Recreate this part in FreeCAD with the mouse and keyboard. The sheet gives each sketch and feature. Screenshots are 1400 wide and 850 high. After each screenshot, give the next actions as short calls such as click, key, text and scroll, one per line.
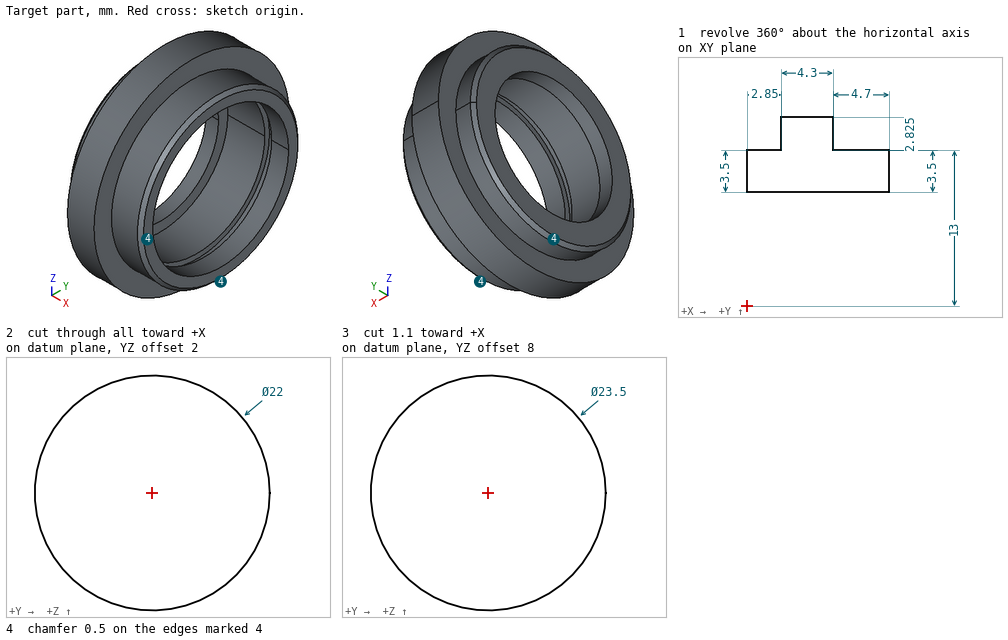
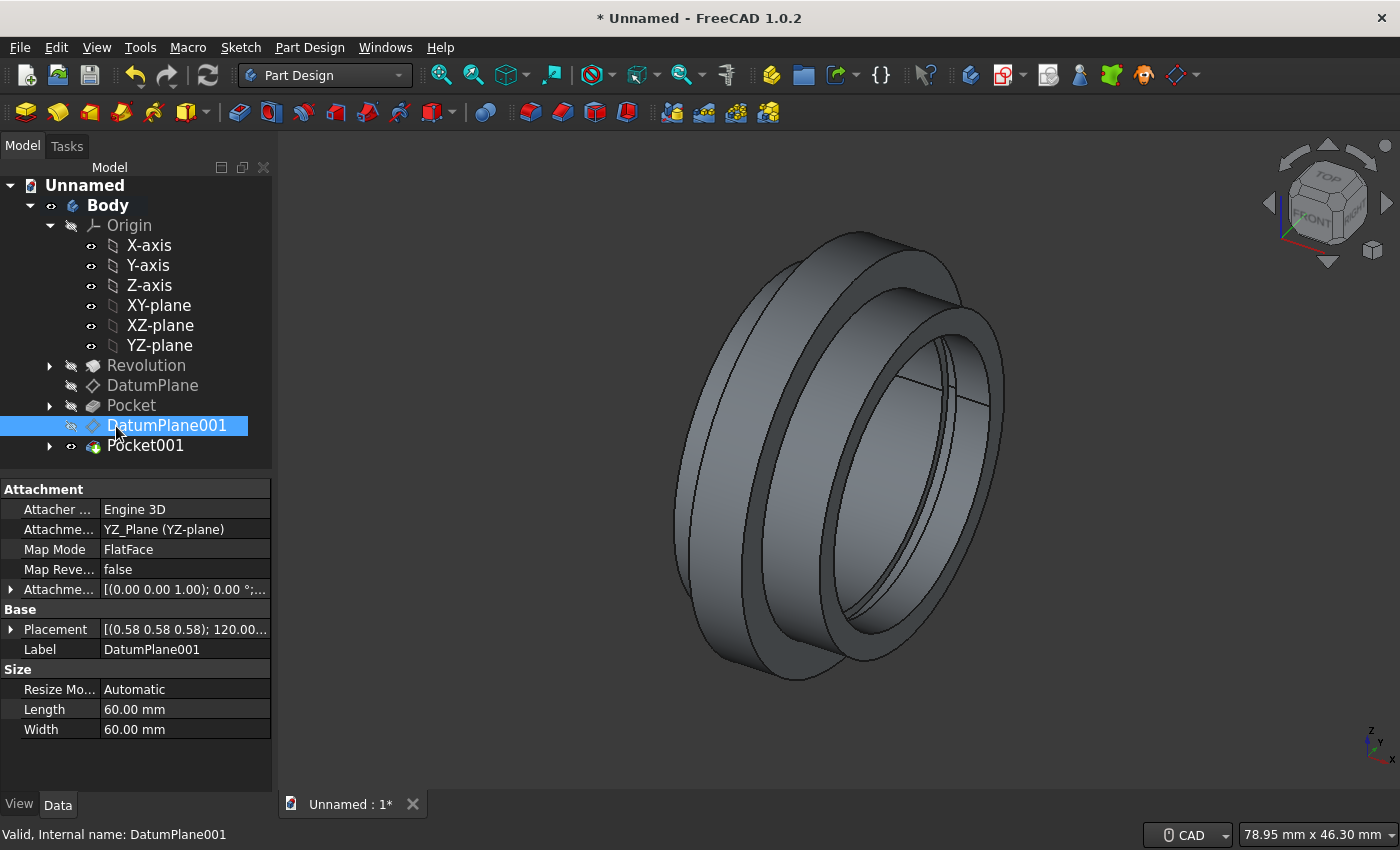
click(820, 575)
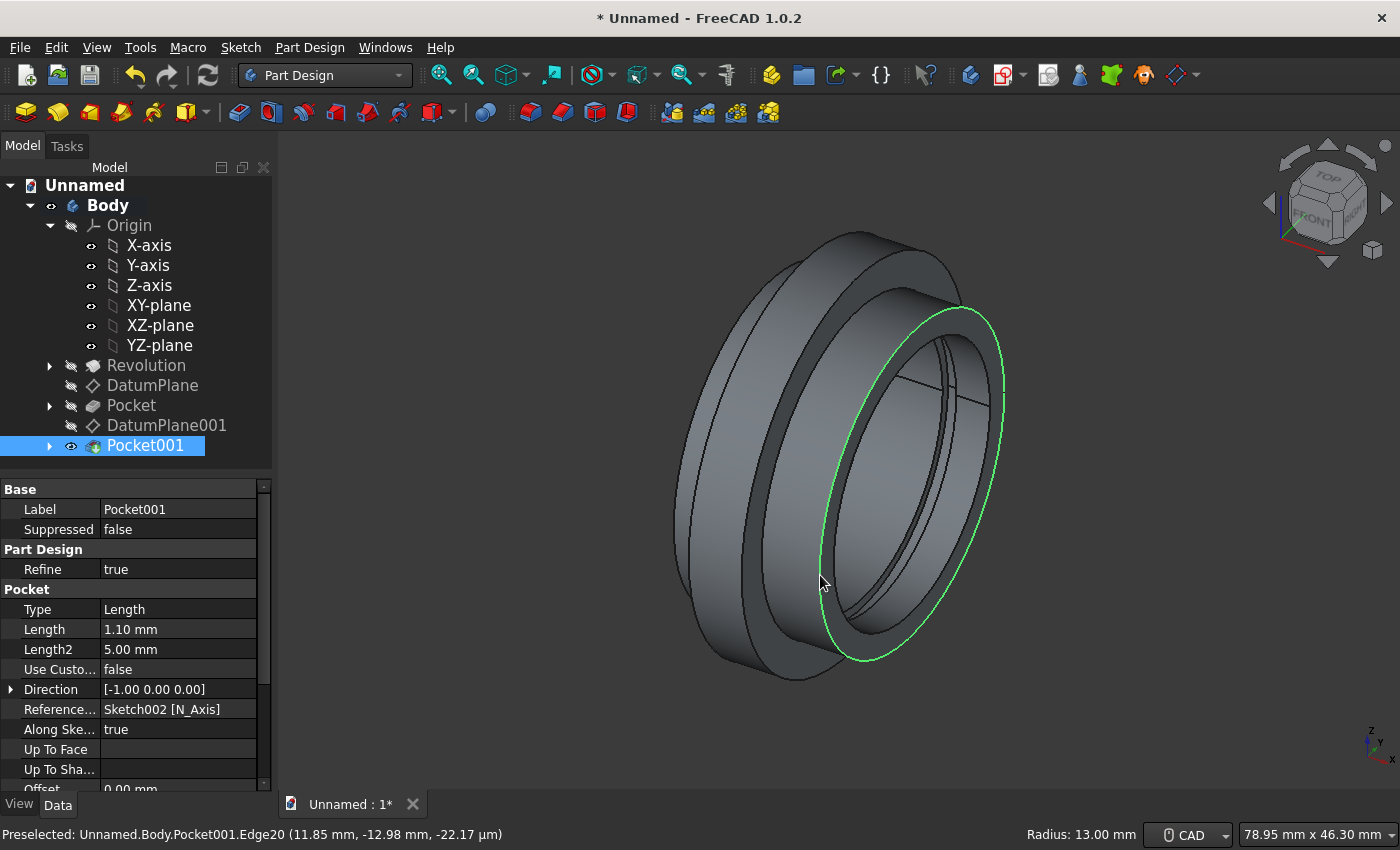
key(0)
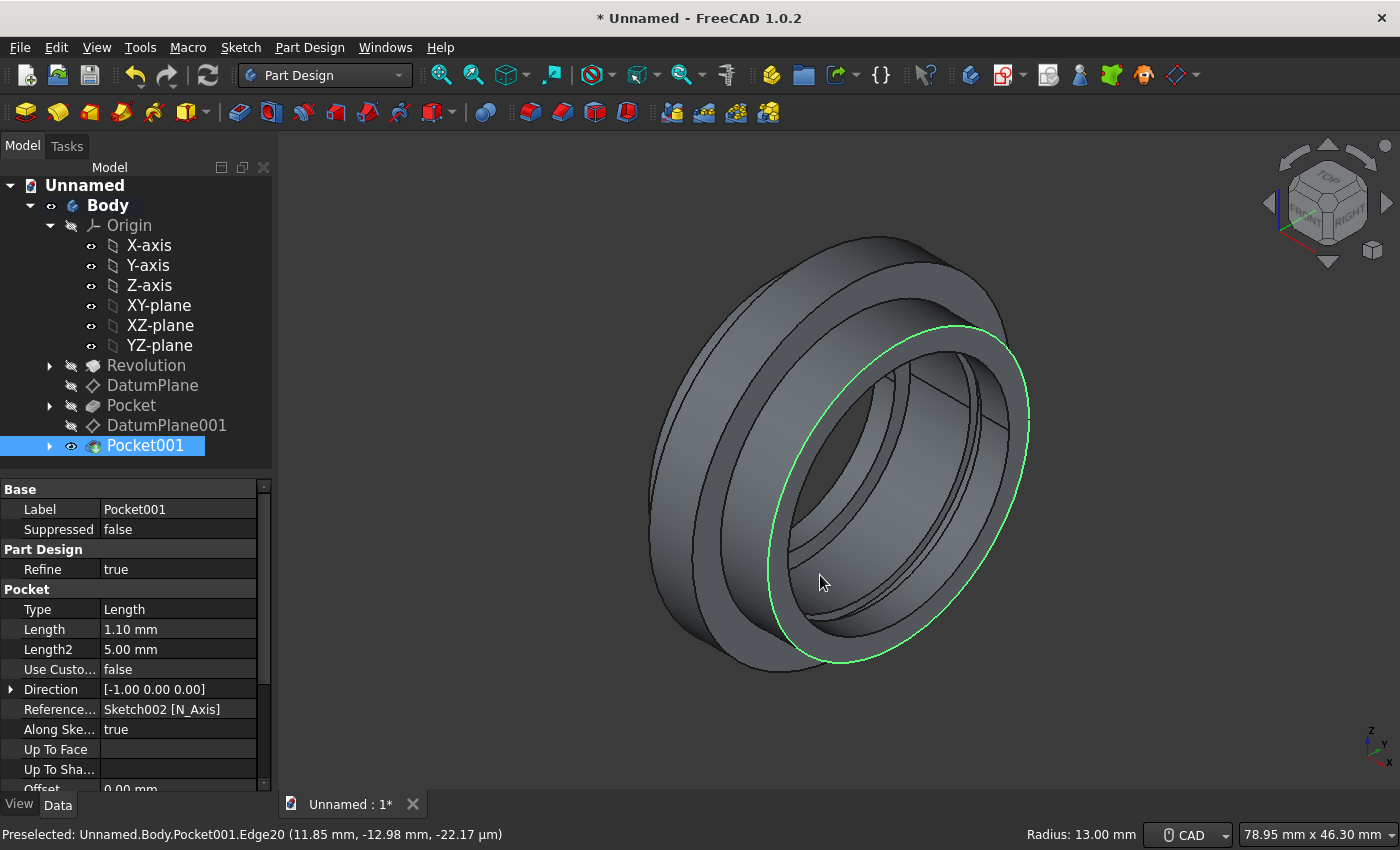
key(2)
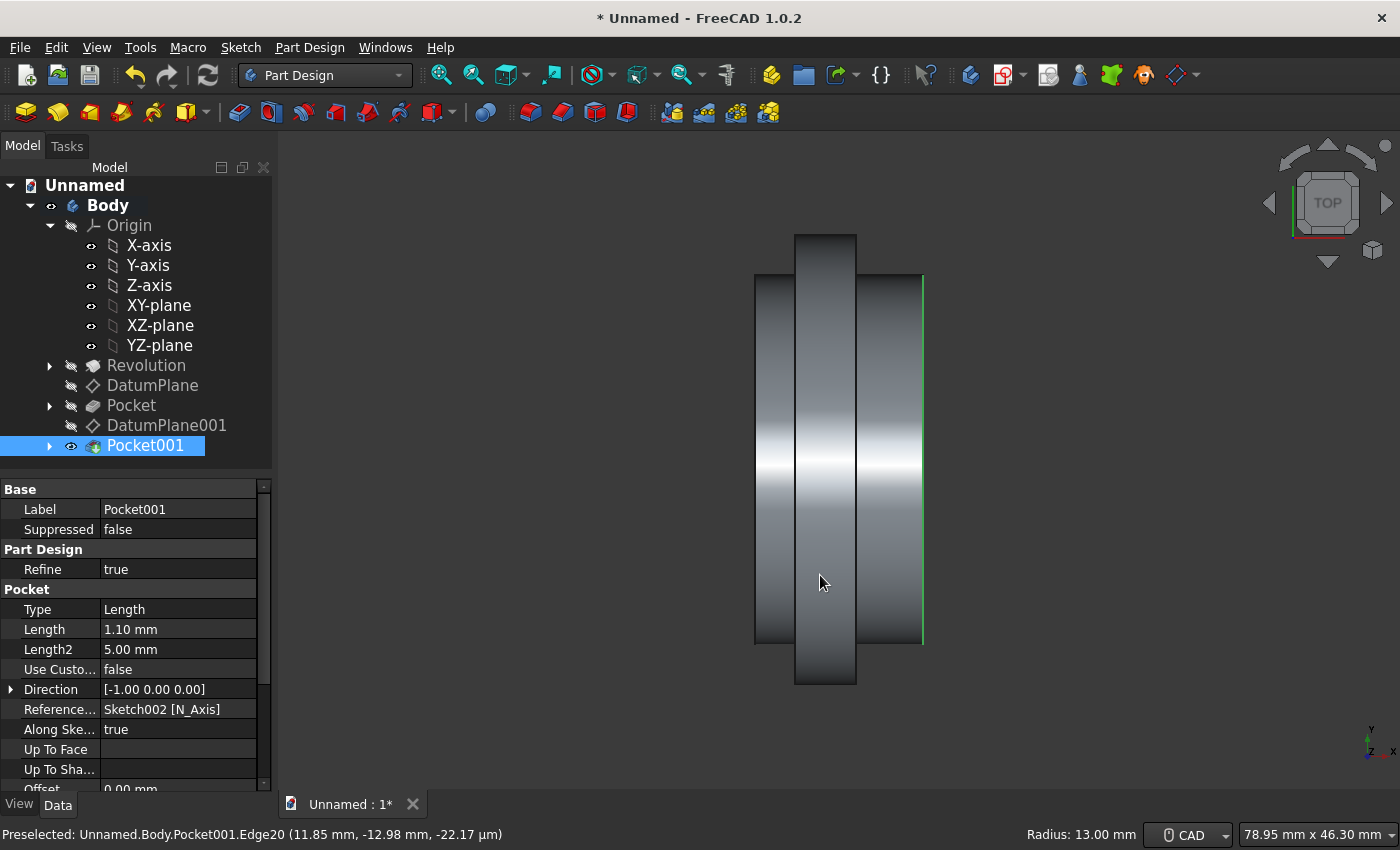
click(755, 608, ctrl)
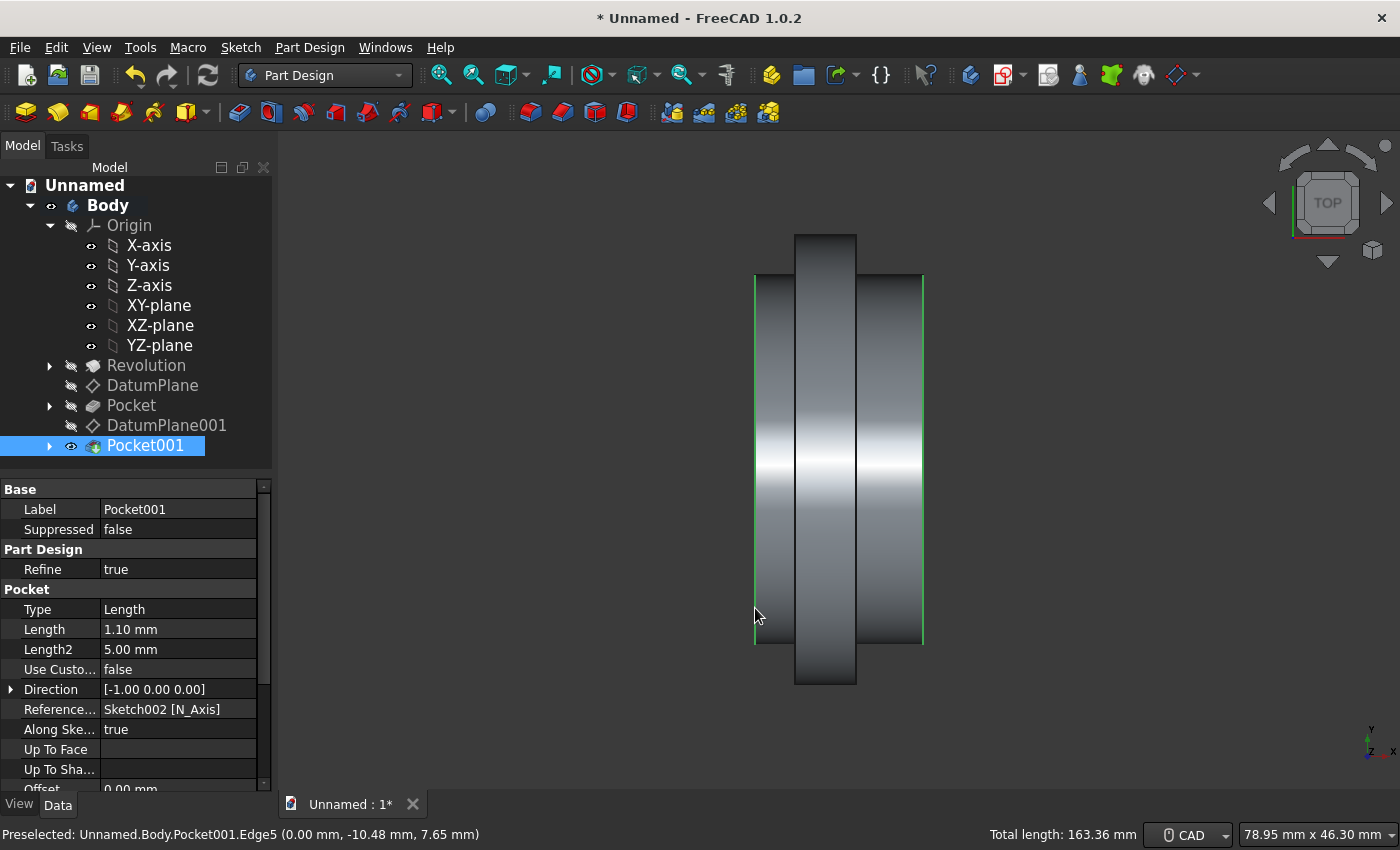
click(564, 112)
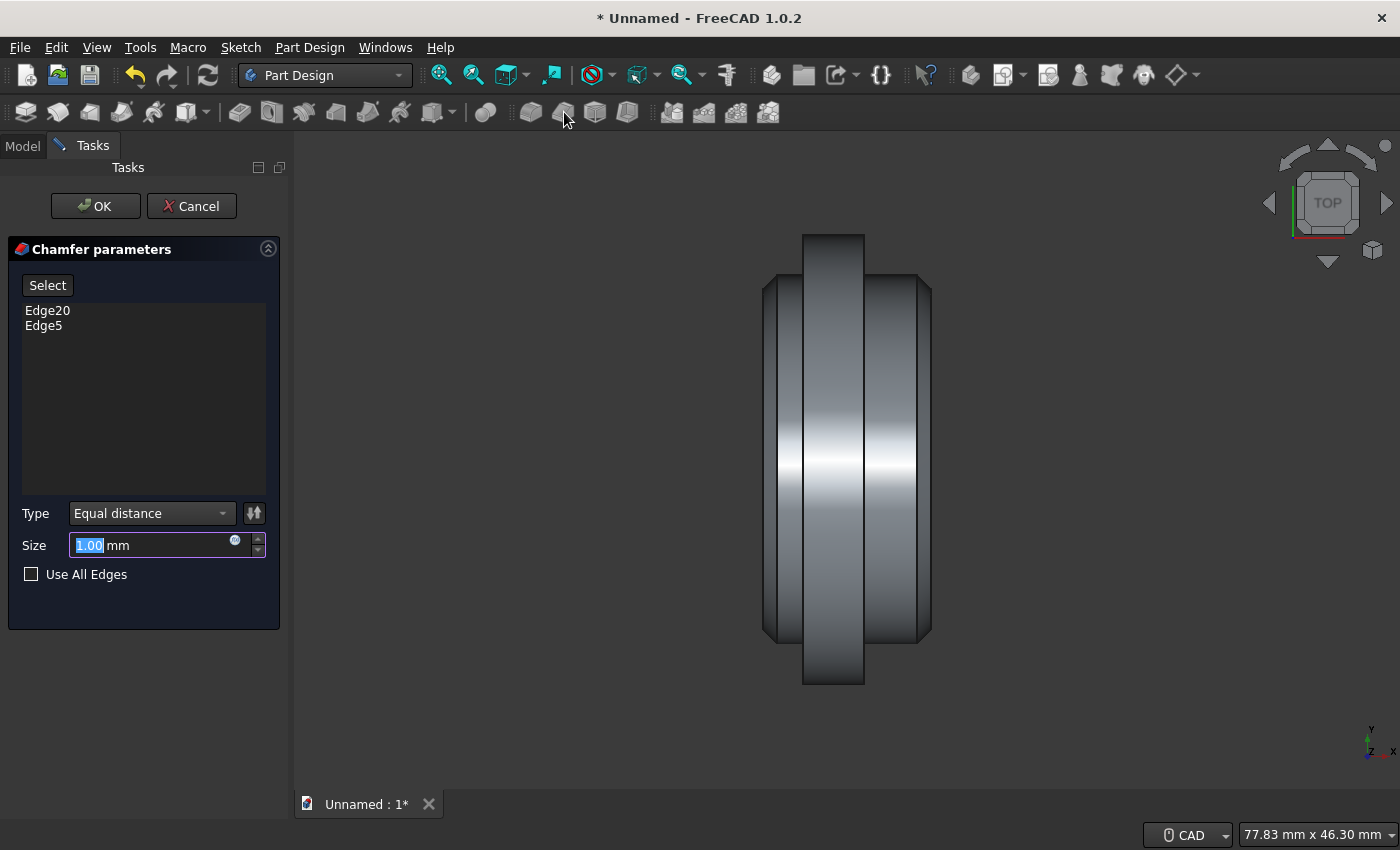
text(0.5)
key(Tab)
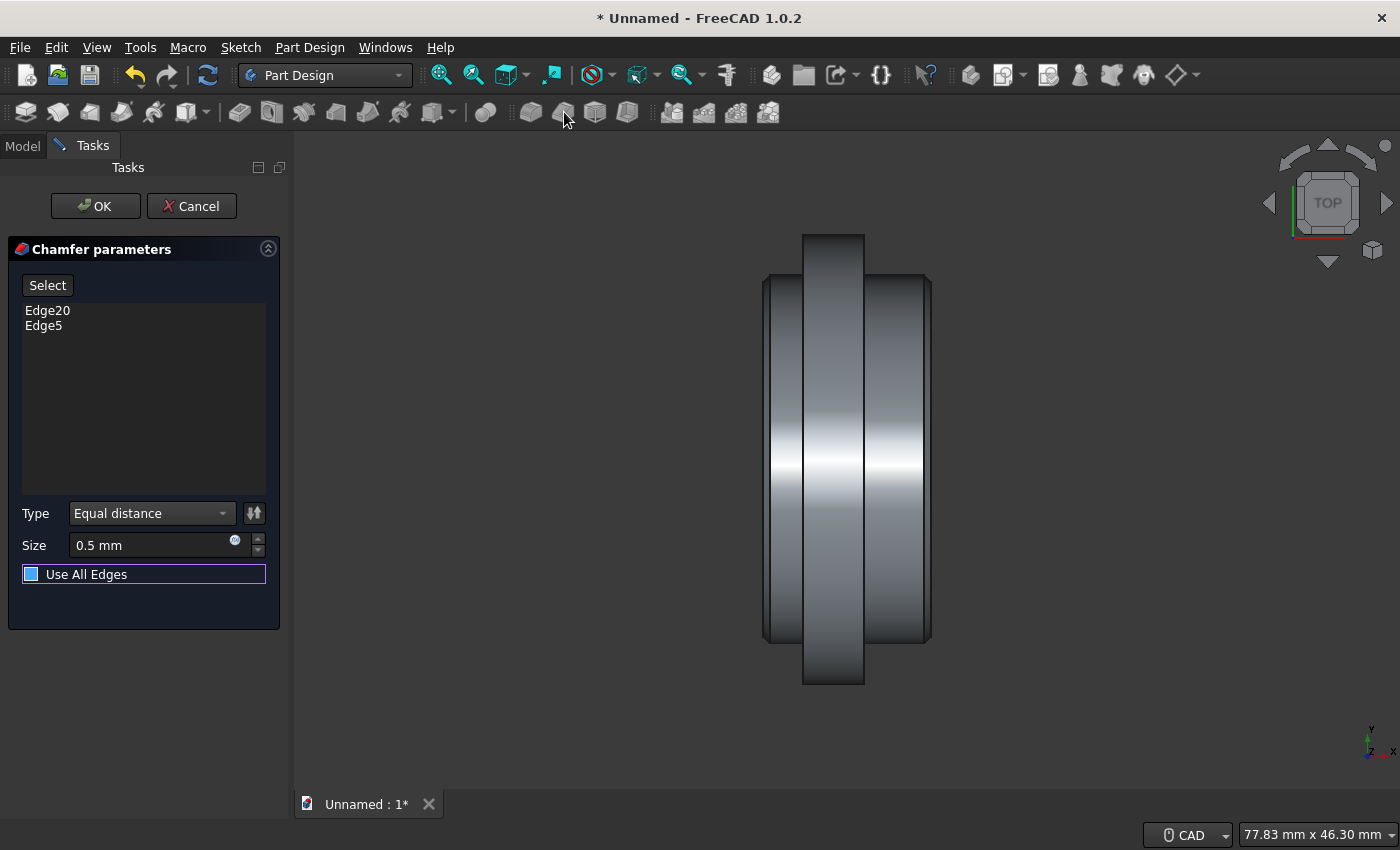
click(96, 206)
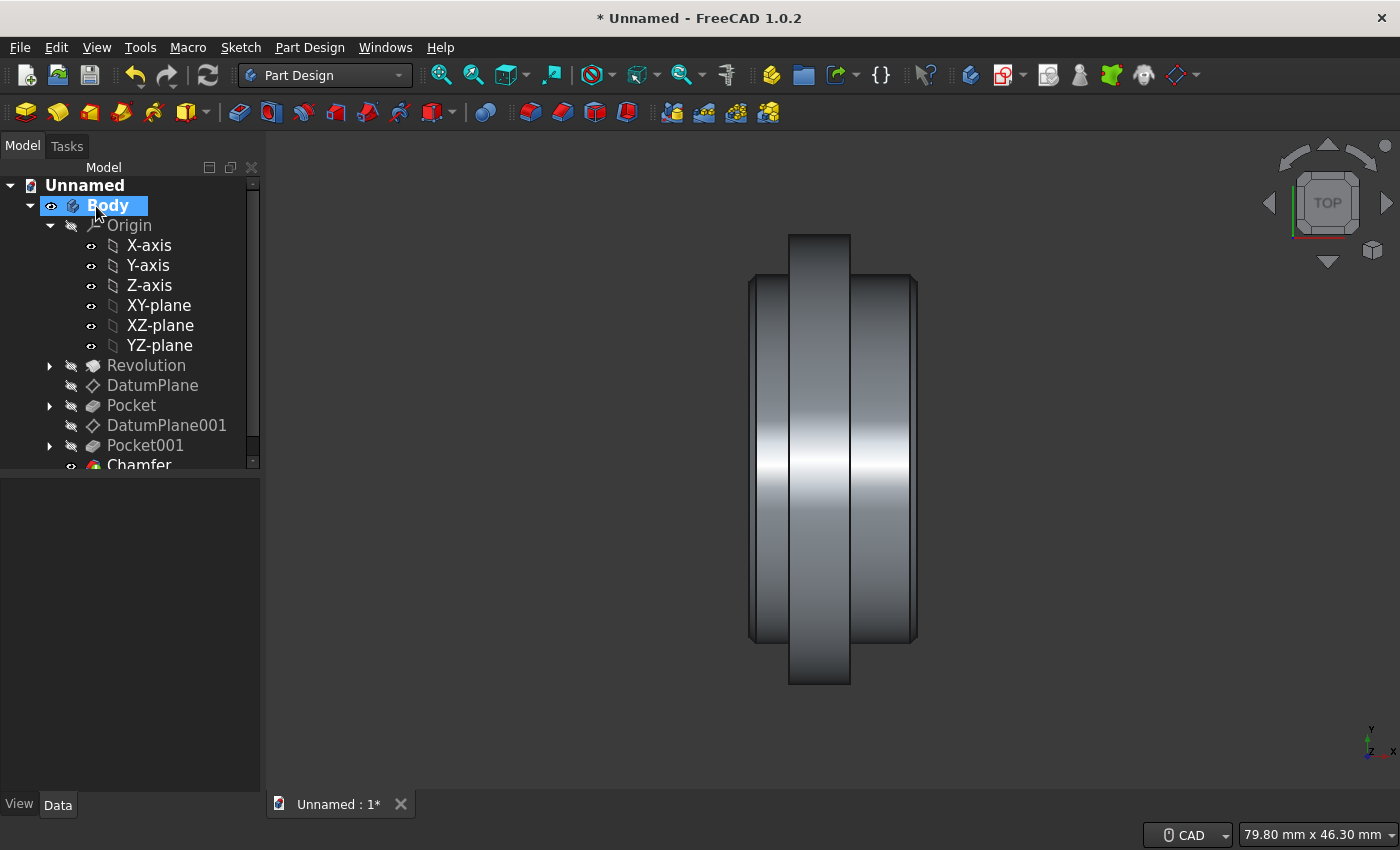
key(0)